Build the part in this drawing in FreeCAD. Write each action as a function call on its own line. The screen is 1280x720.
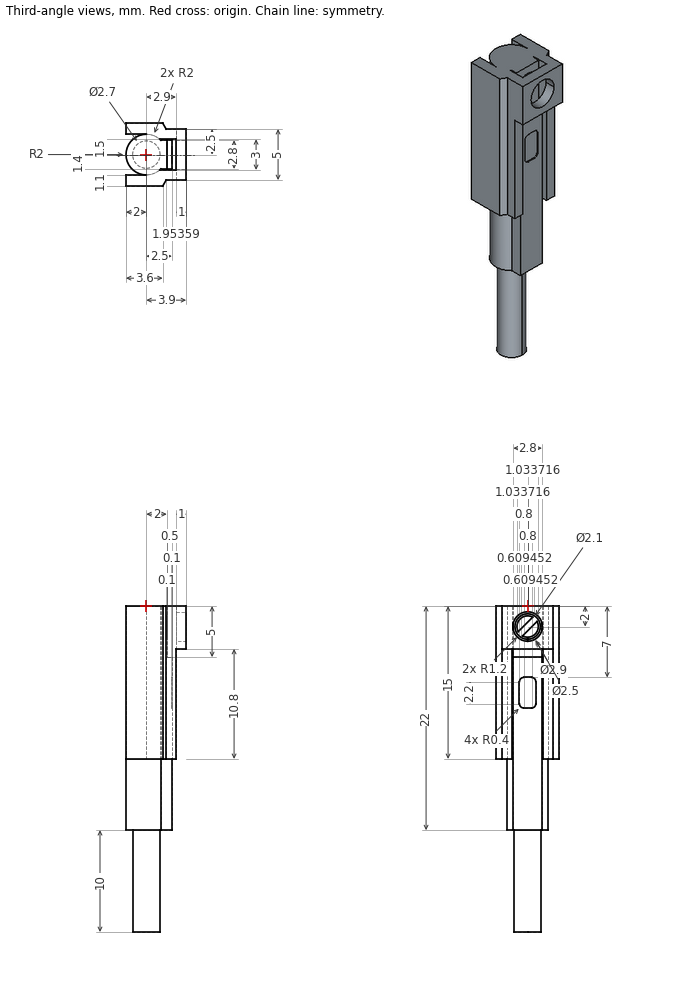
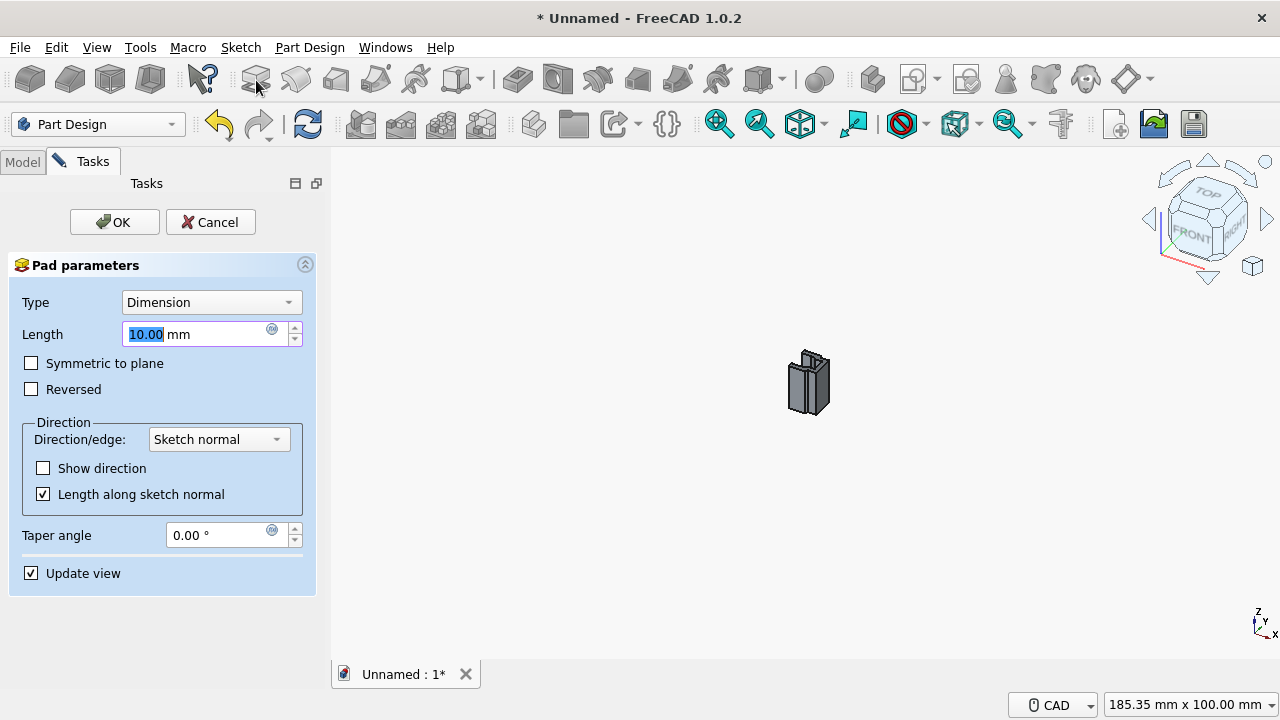
text(15)
key(Tab)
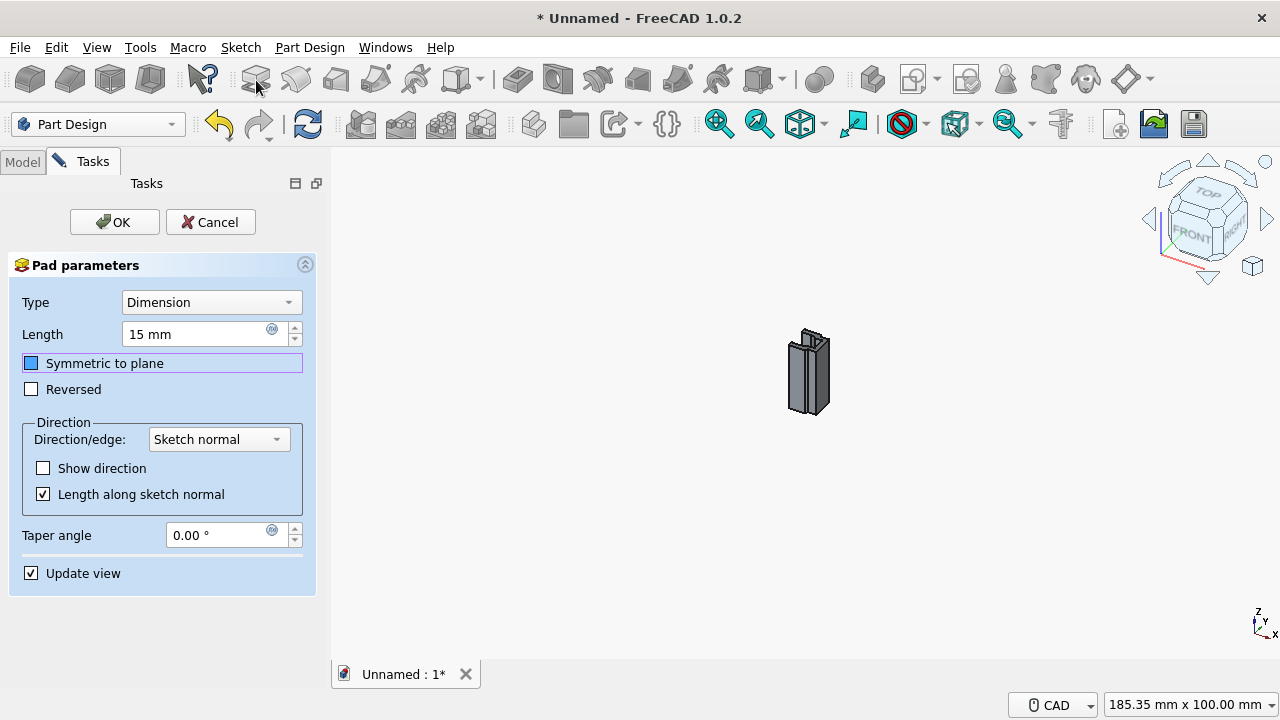
click(30, 389)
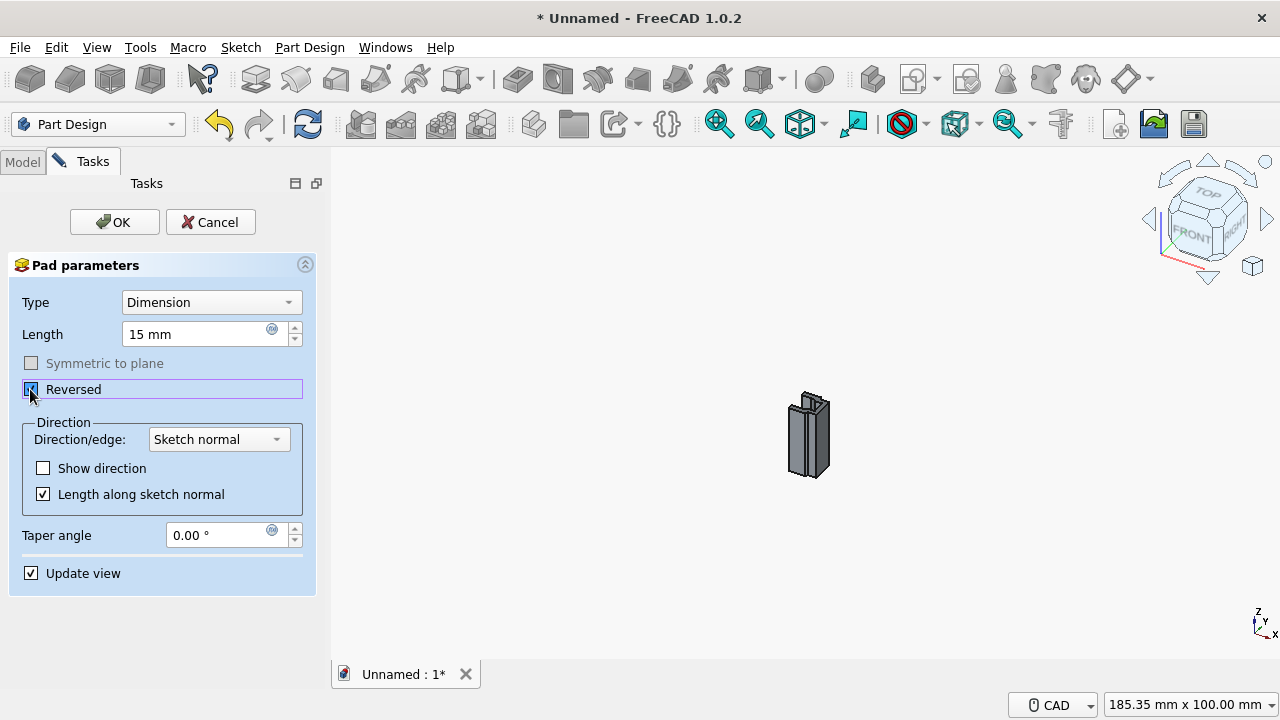
click(115, 222)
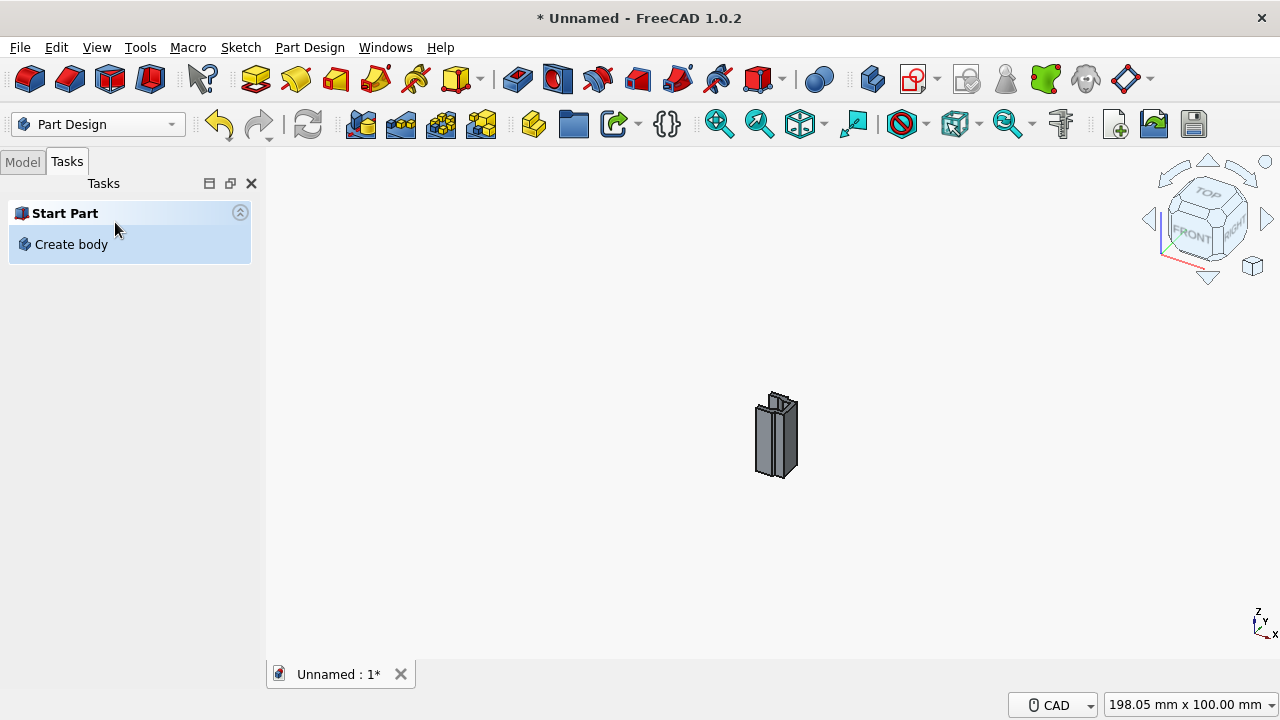
click(720, 124)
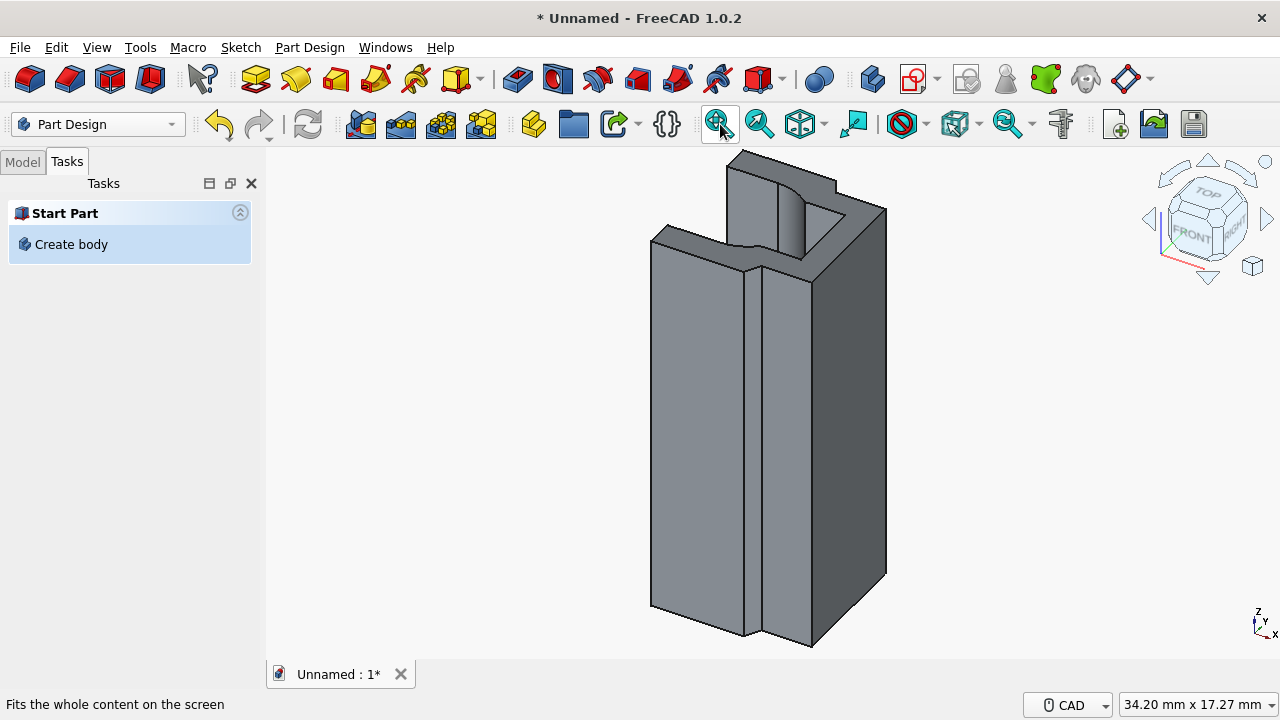
click(23, 161)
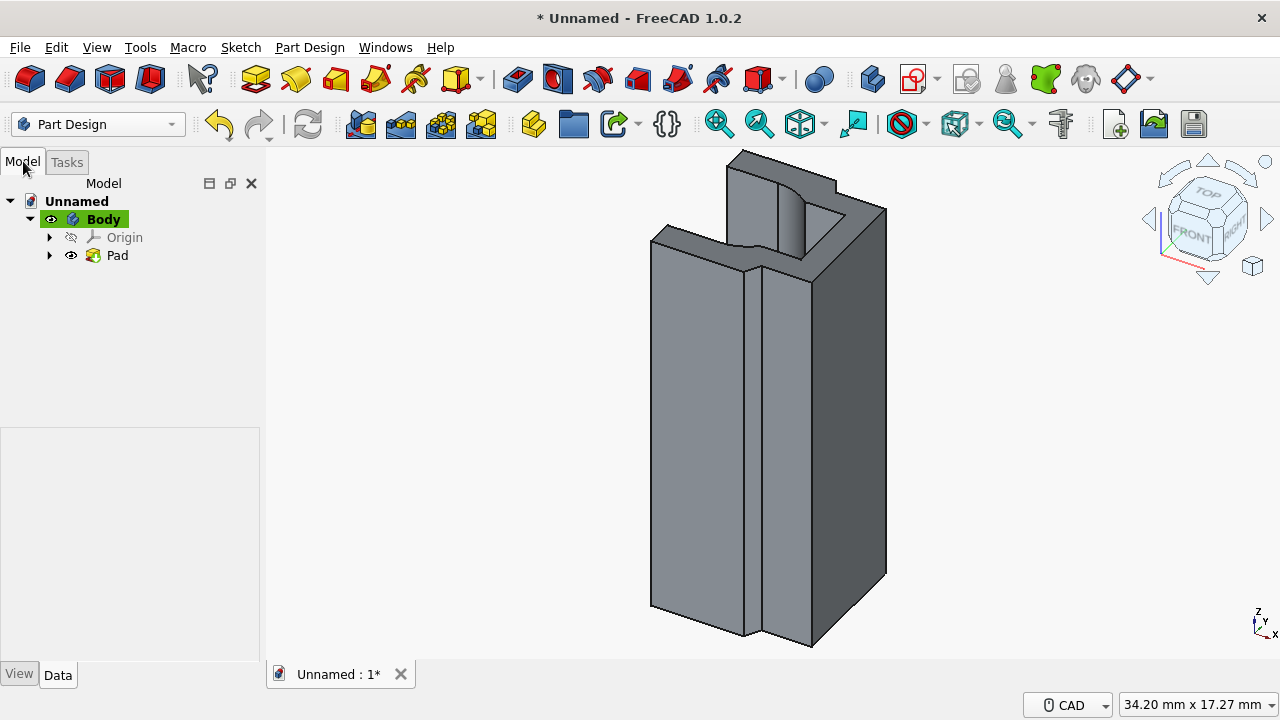
click(50, 237)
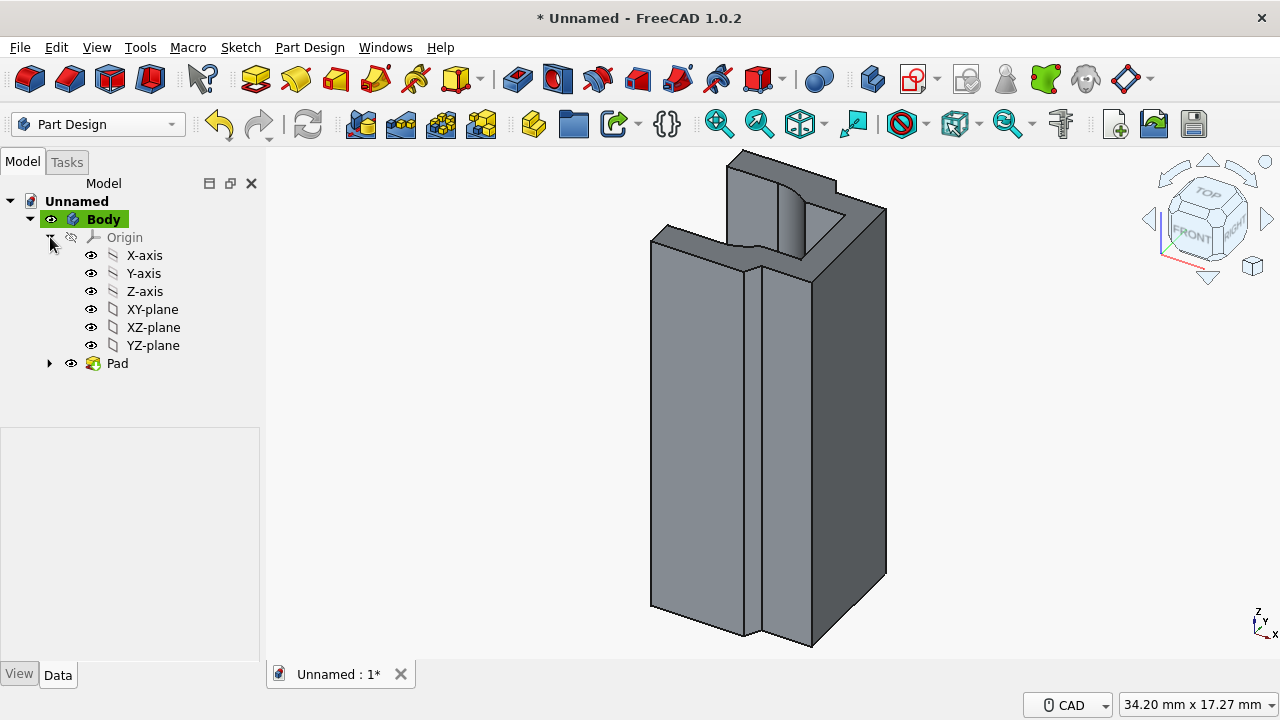
click(136, 309)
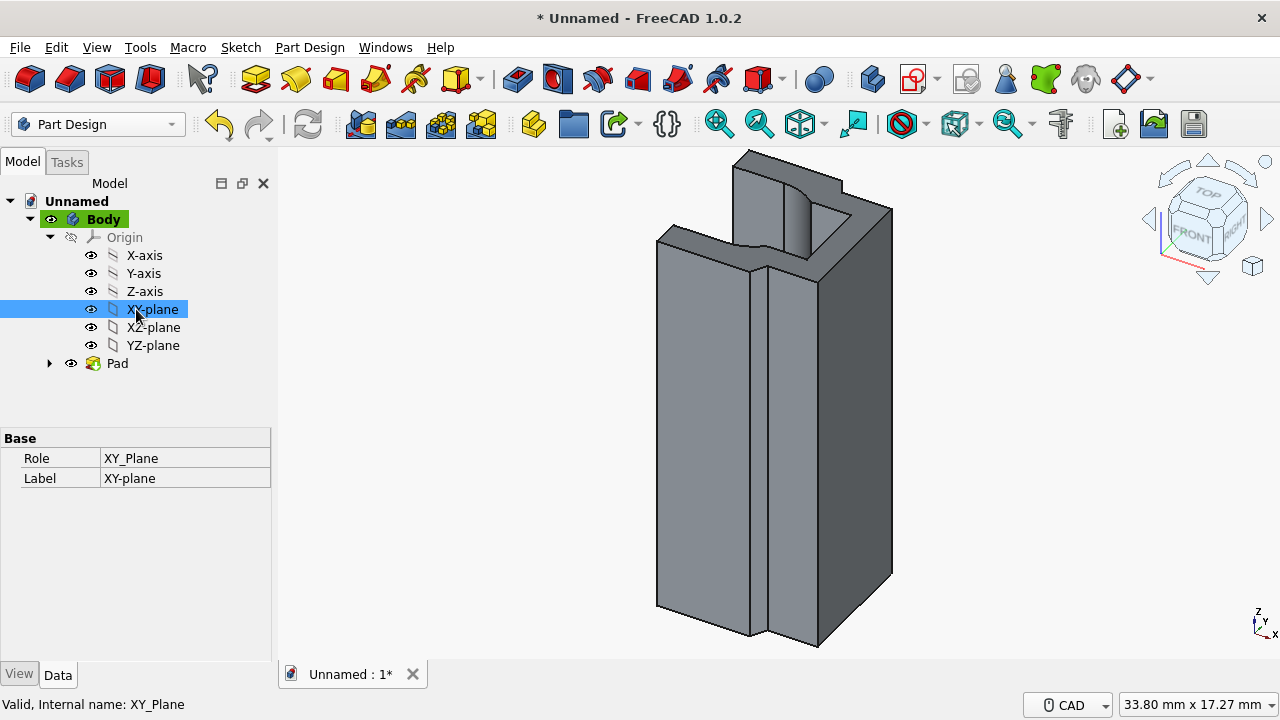
click(1126, 80)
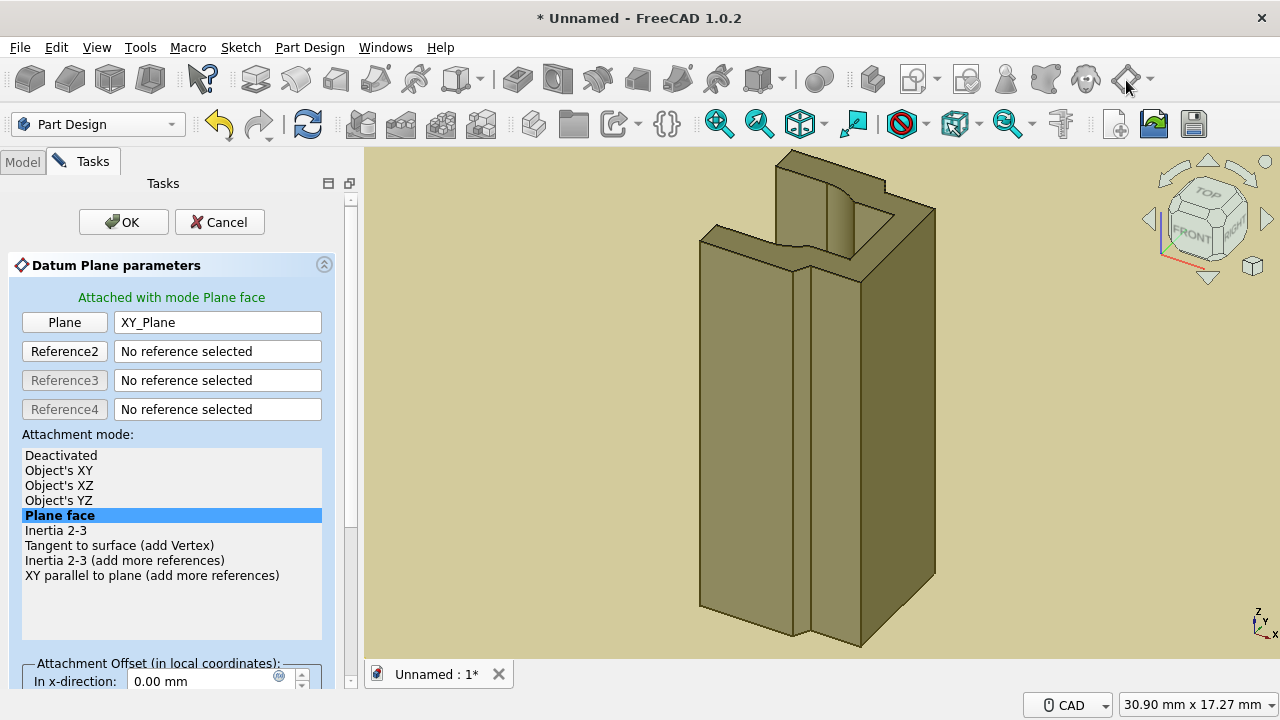
scroll(351, 440, down, 3)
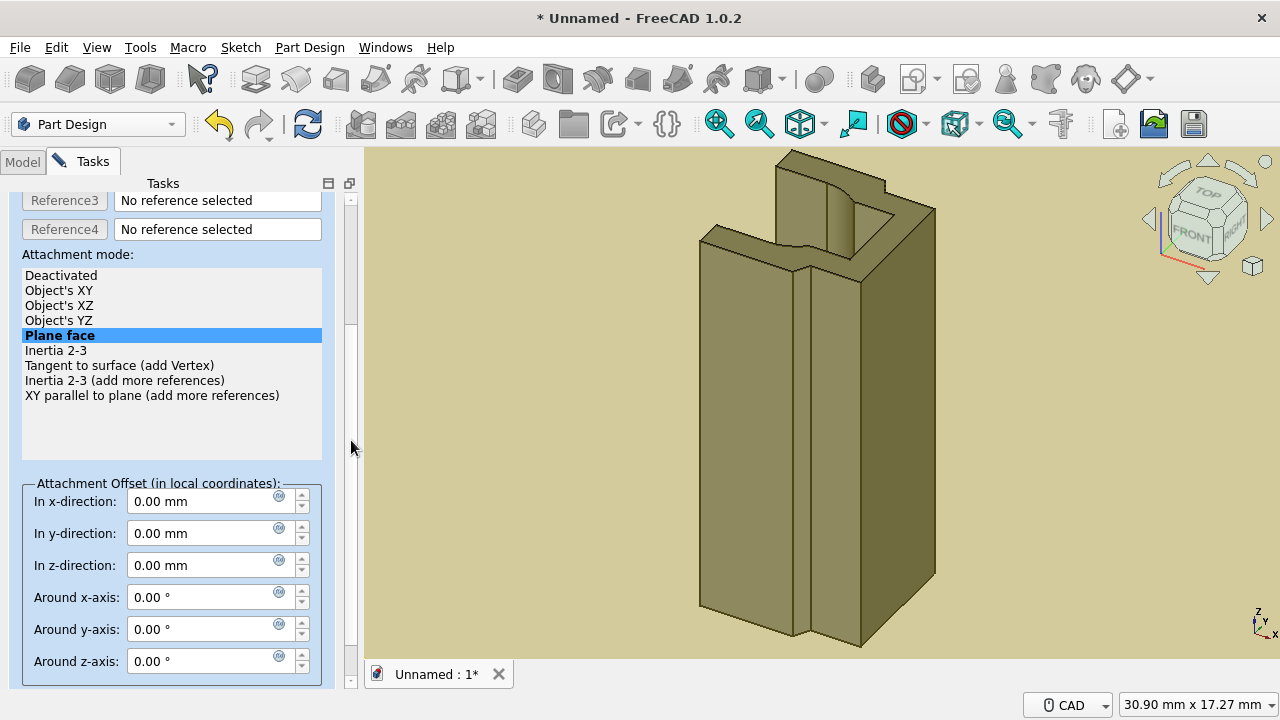
triple_click(210, 565)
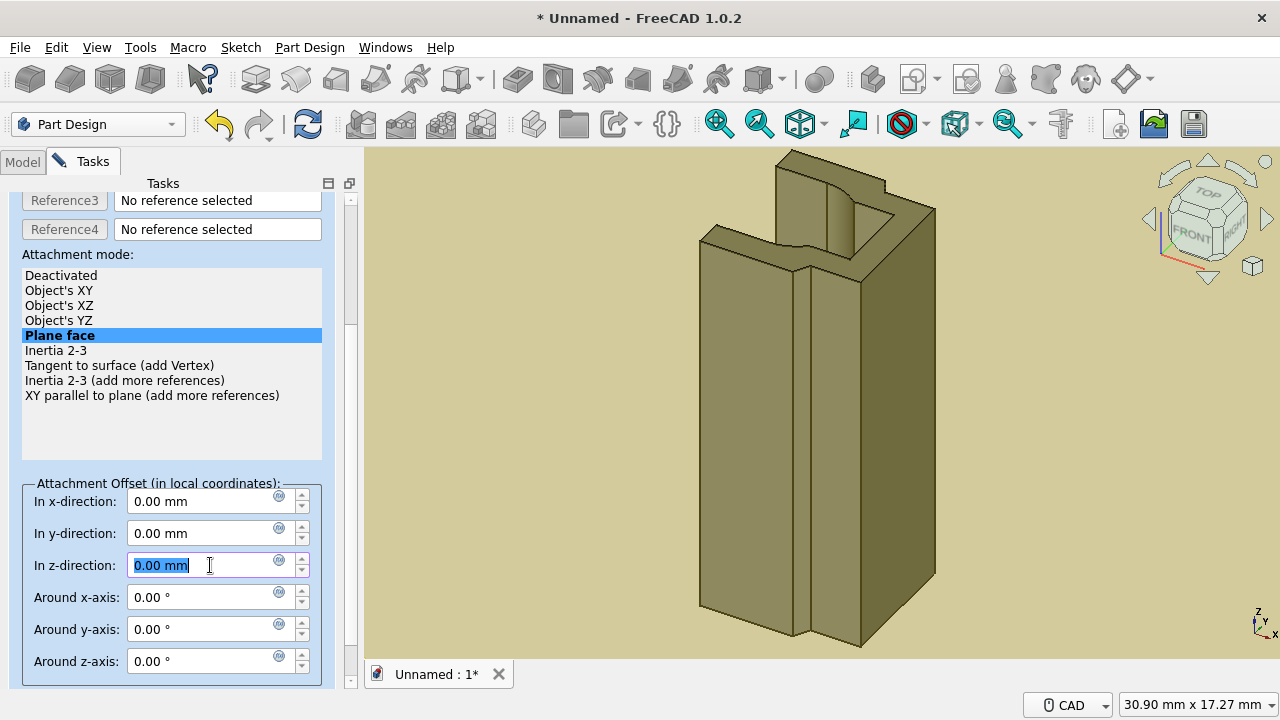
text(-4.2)
key(Tab)